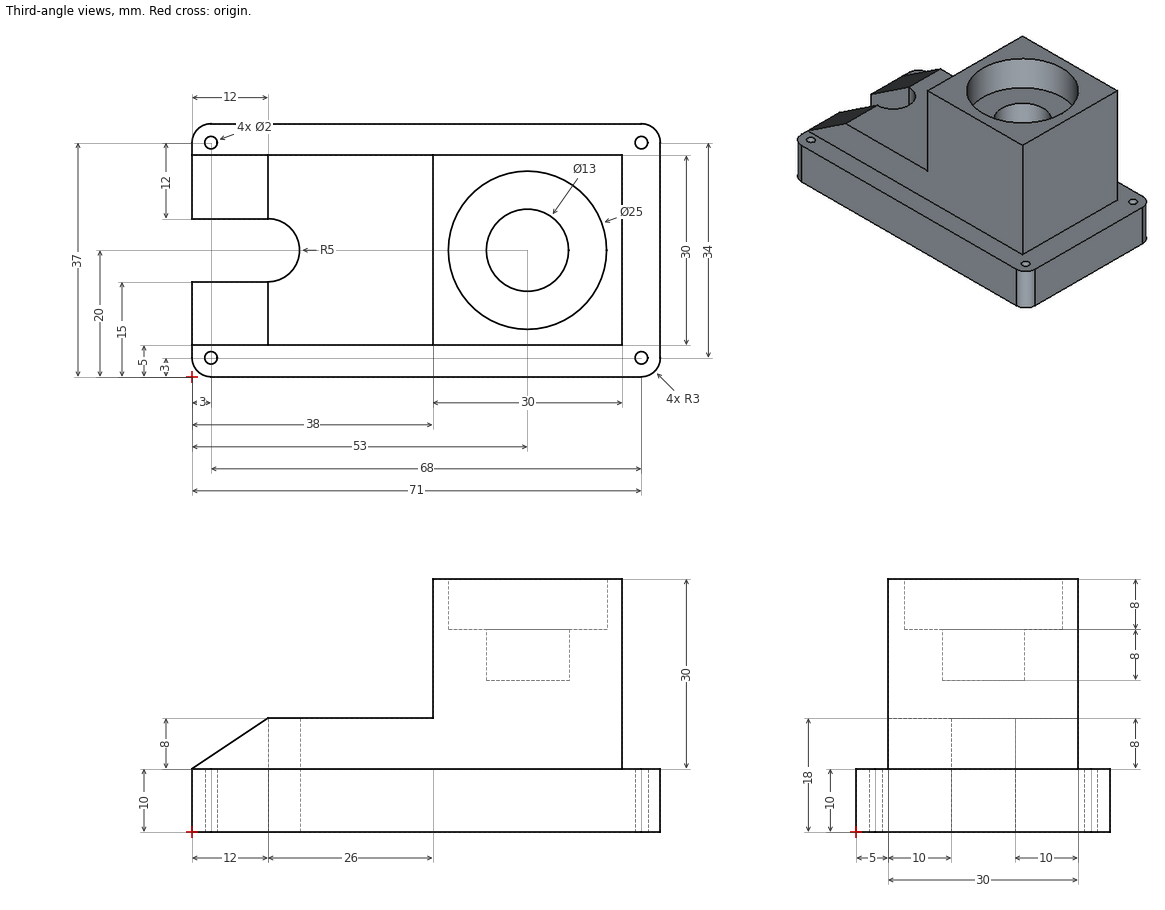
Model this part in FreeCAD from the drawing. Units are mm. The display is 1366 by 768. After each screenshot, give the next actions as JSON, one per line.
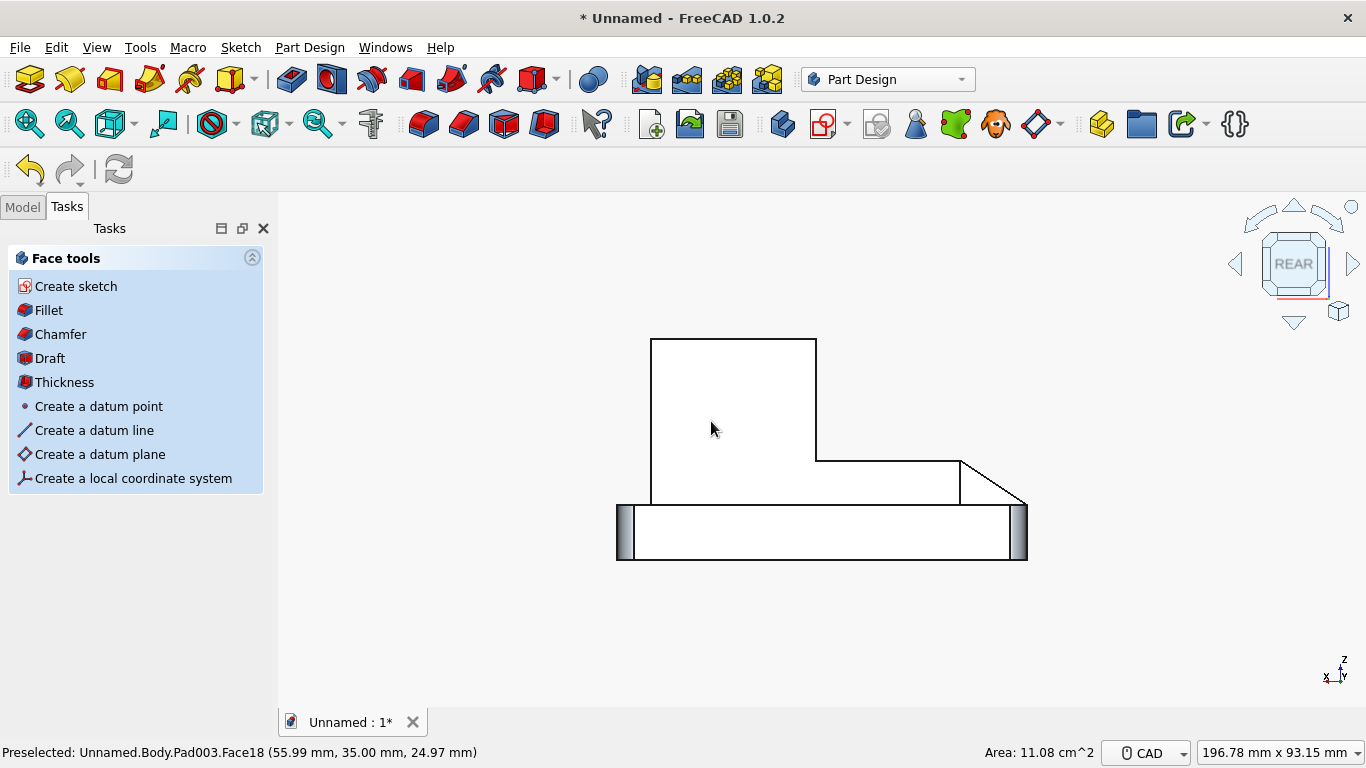
{"action": "left_click", "coordinate": [824, 124]}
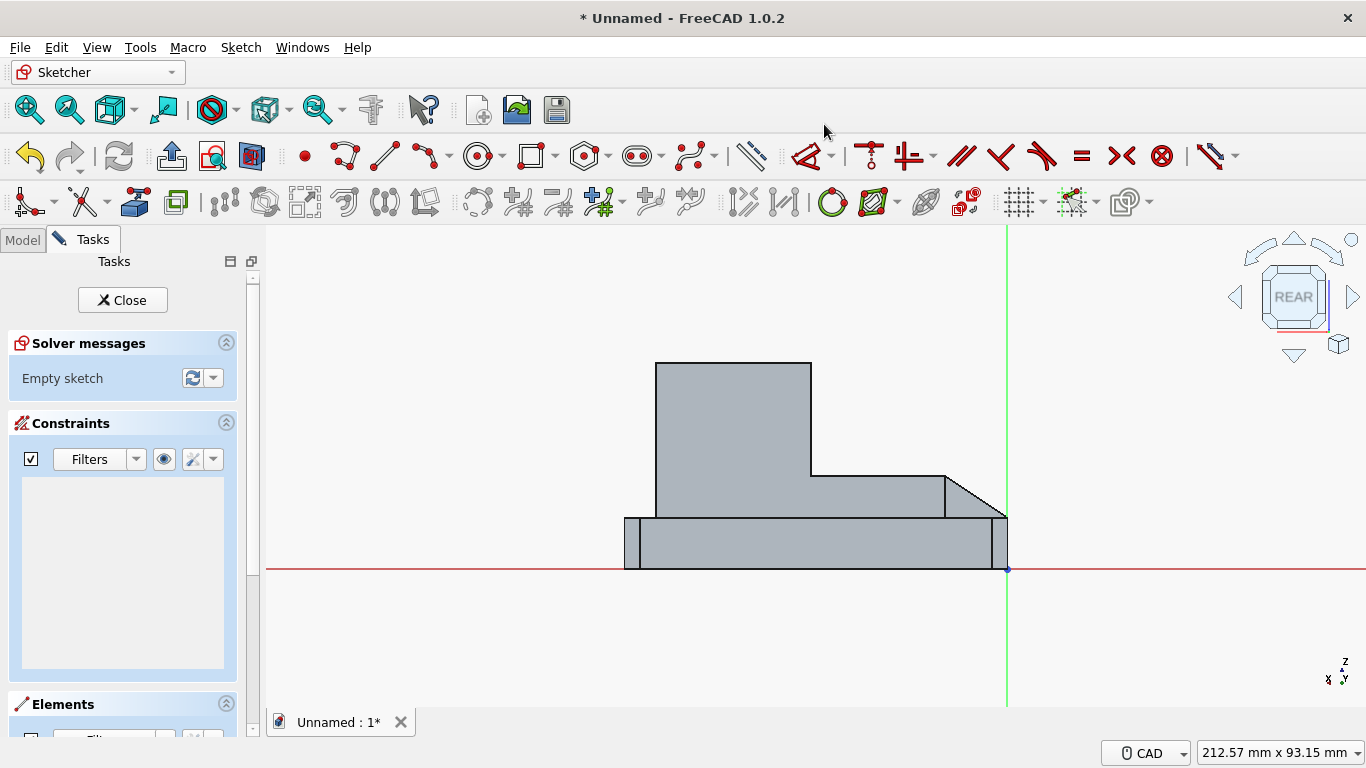
{"action": "left_click", "coordinate": [252, 156]}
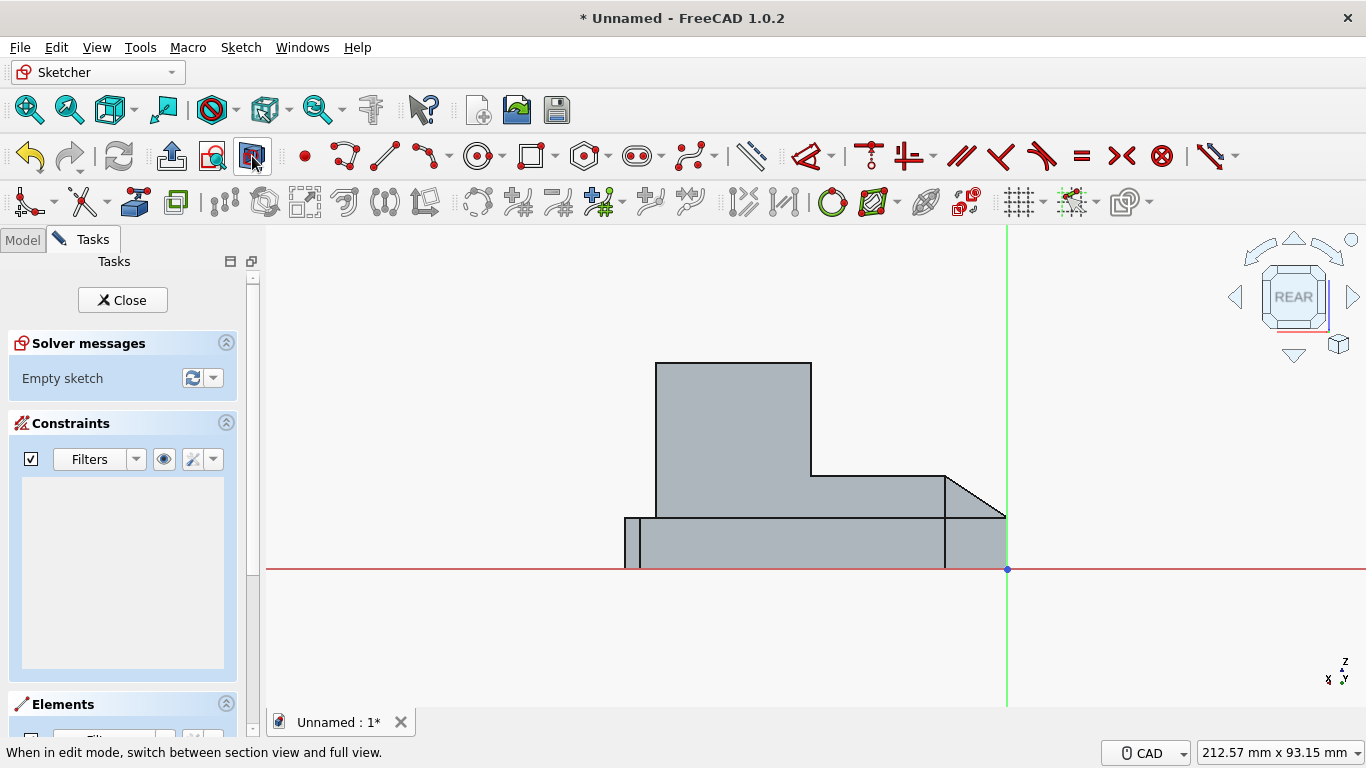
{"action": "scroll", "coordinate": [1075, 547], "scroll_direction": "up", "scroll_amount": 6}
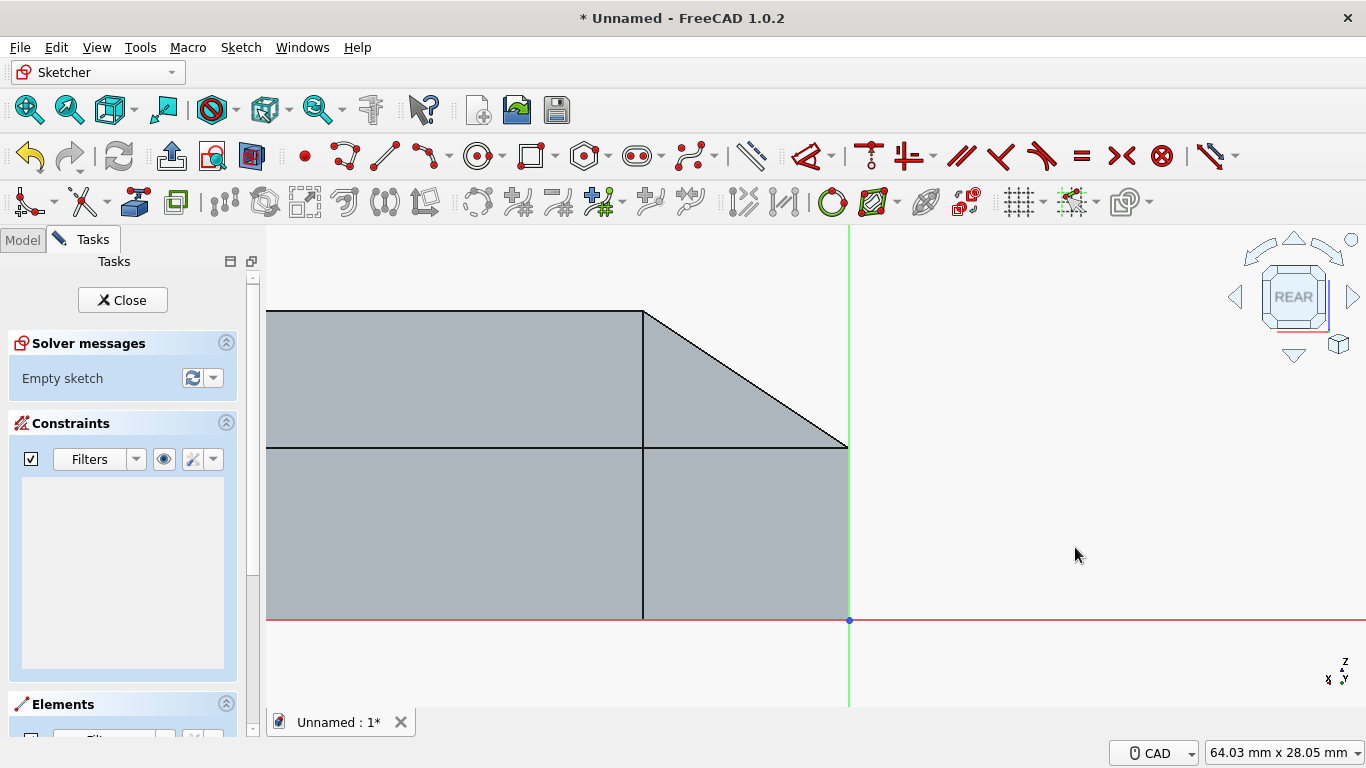
{"action": "left_click", "coordinate": [346, 156]}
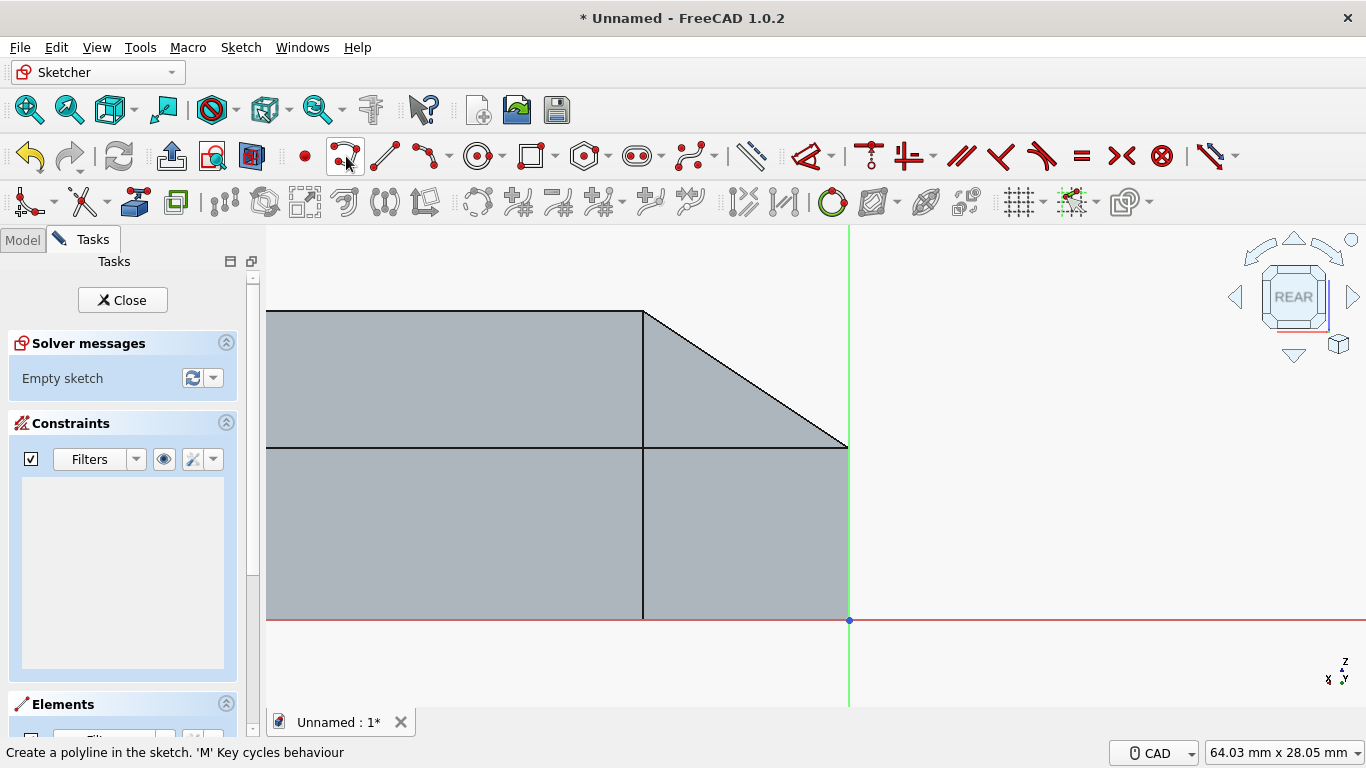
{"action": "left_click", "coordinate": [849, 448]}
{"action": "left_click", "coordinate": [643, 311]}
{"action": "left_click", "coordinate": [643, 448]}
{"action": "left_click", "coordinate": [849, 449]}
{"action": "key", "text": "Escape"}
{"action": "key", "text": "Escape"}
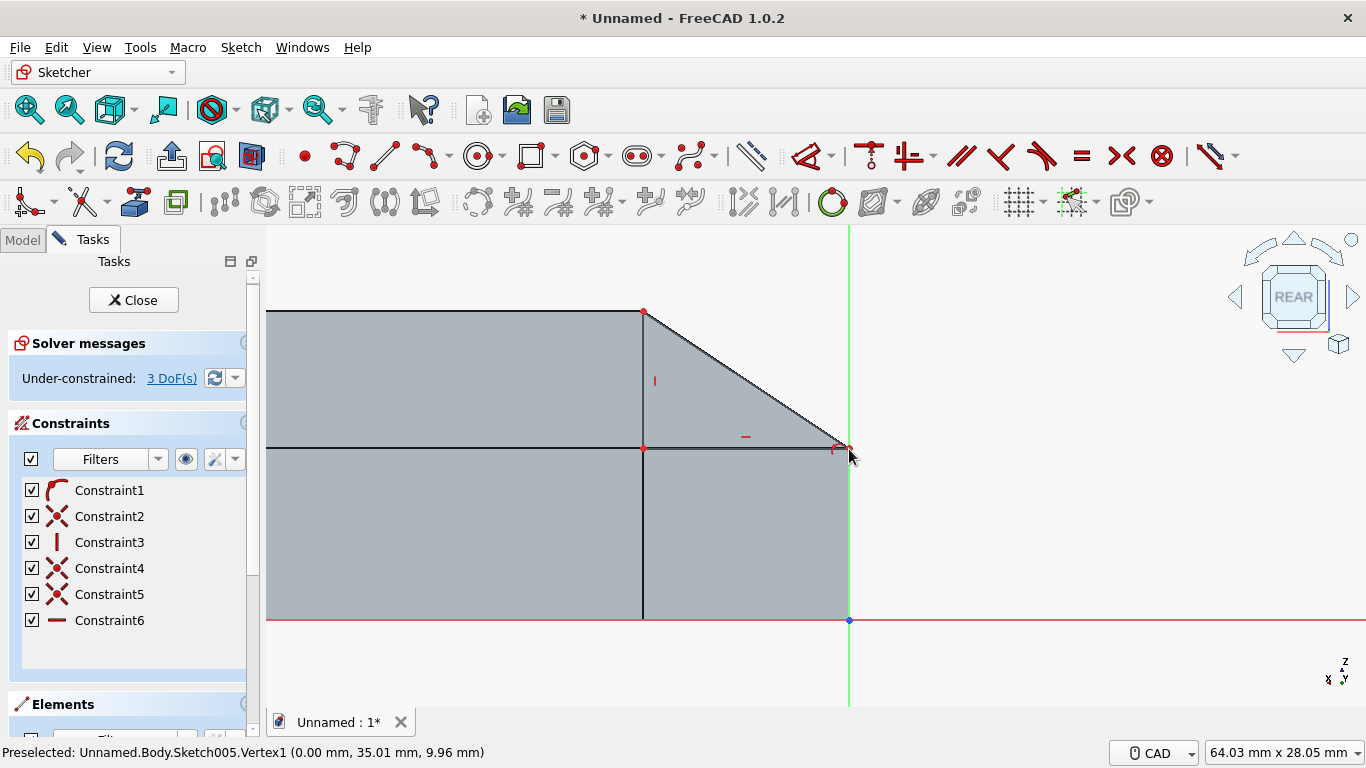
{"action": "left_click", "coordinate": [806, 156]}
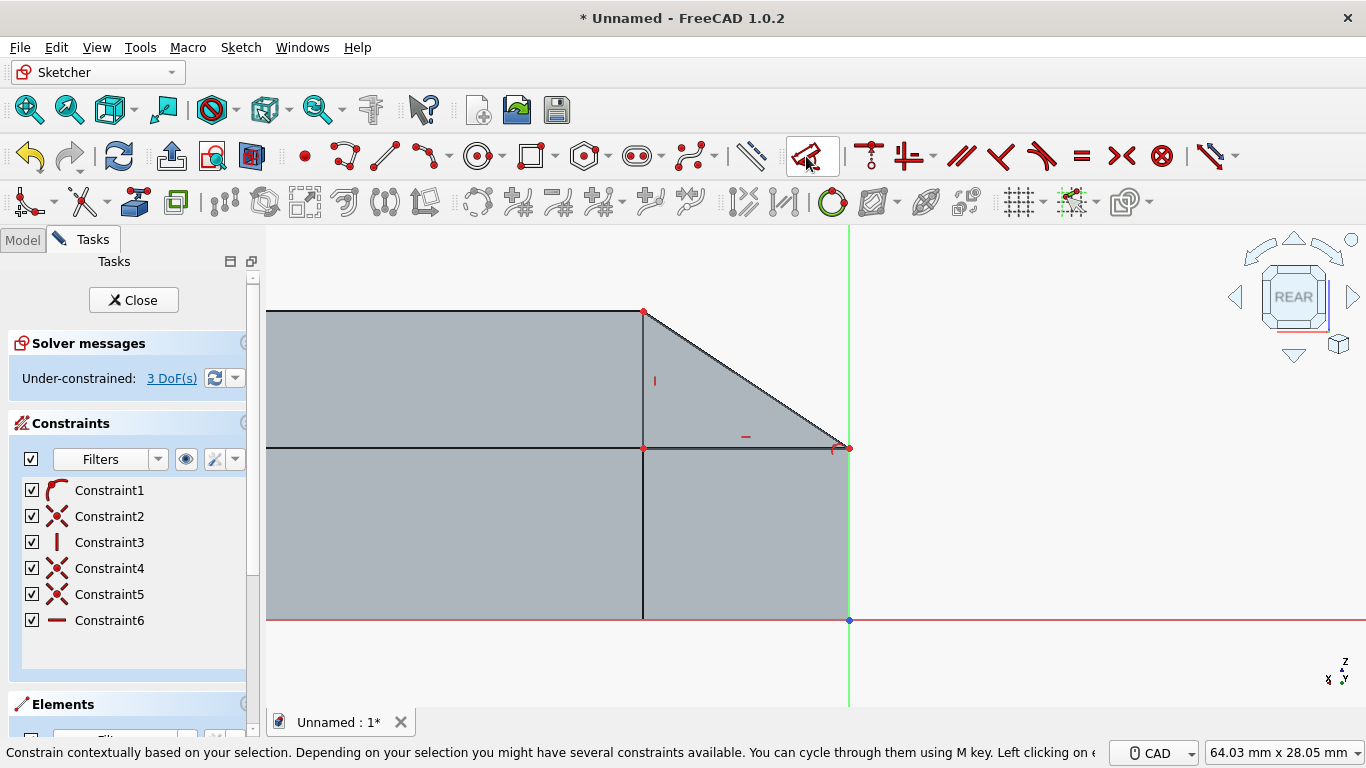
{"action": "left_click", "coordinate": [643, 353]}
{"action": "left_click", "coordinate": [609, 380]}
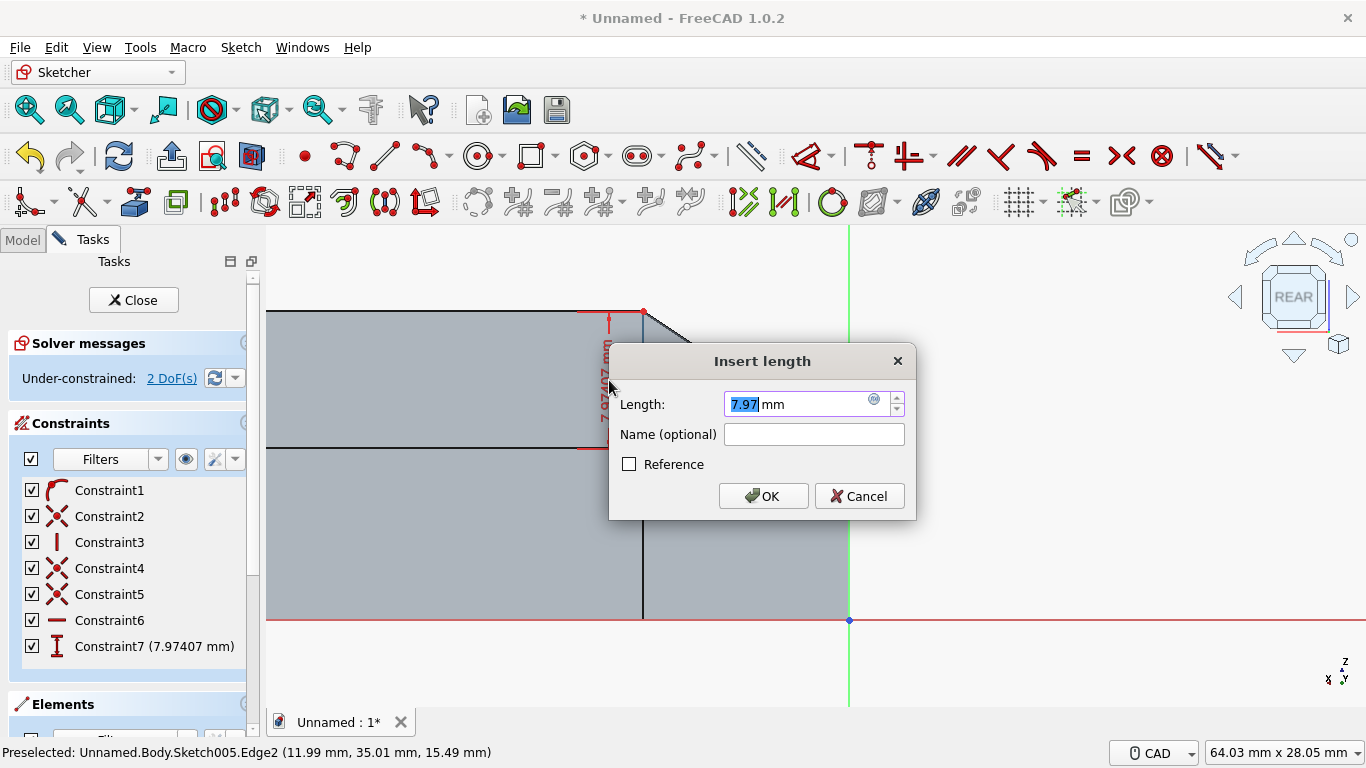
{"action": "type", "text": "8"}
{"action": "key", "text": "Return"}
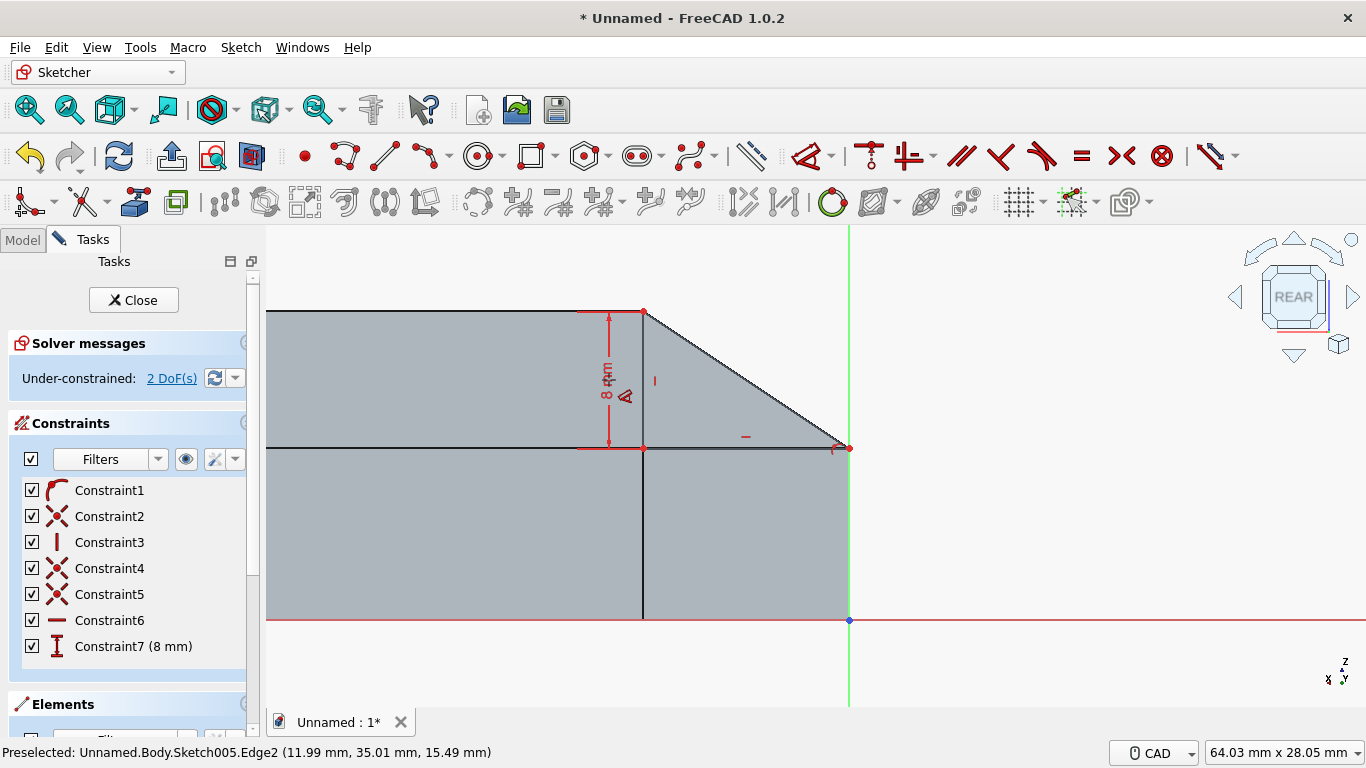
{"action": "left_click", "coordinate": [705, 449]}
{"action": "left_click", "coordinate": [746, 415]}